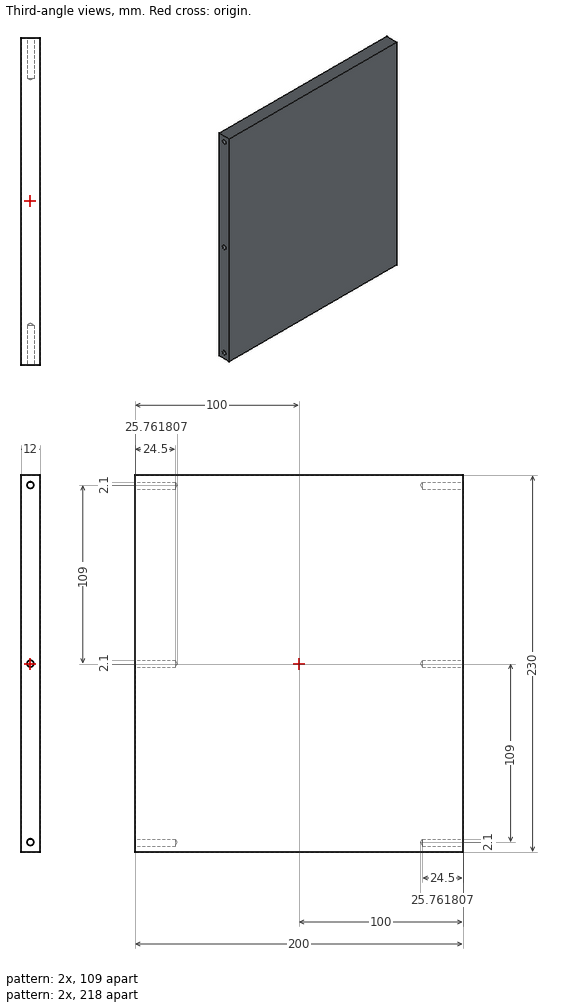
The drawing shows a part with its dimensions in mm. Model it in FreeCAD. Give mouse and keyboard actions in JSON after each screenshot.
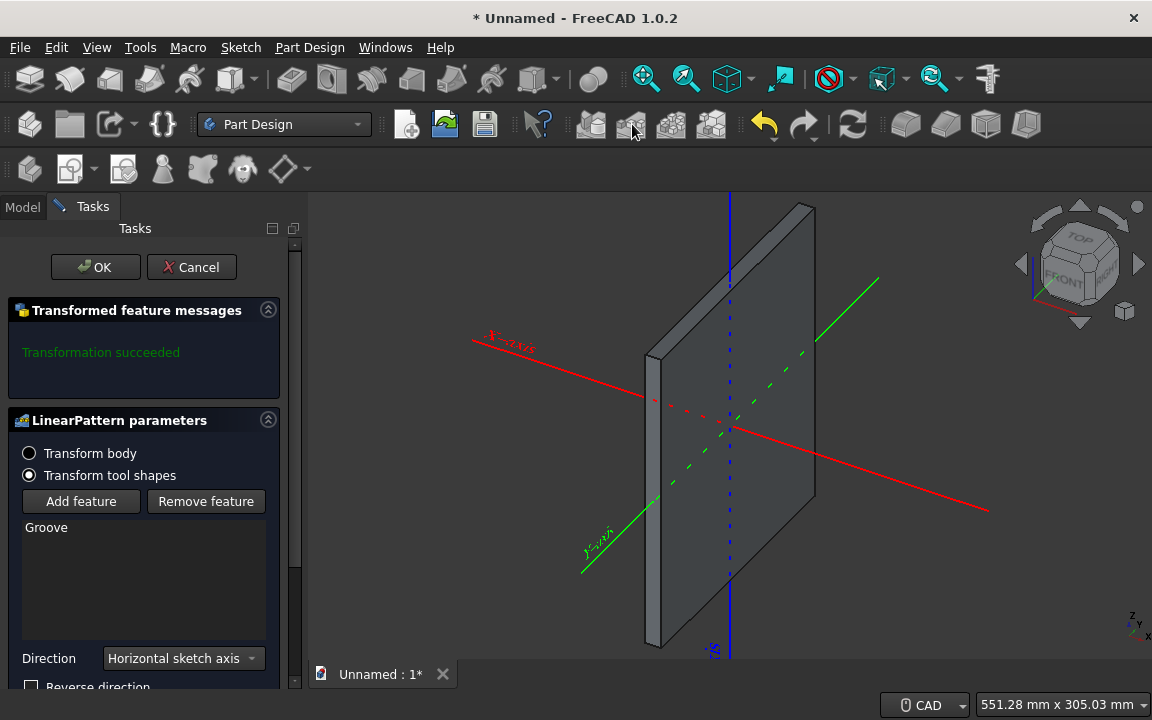
{"action": "left_click", "coordinate": [184, 658]}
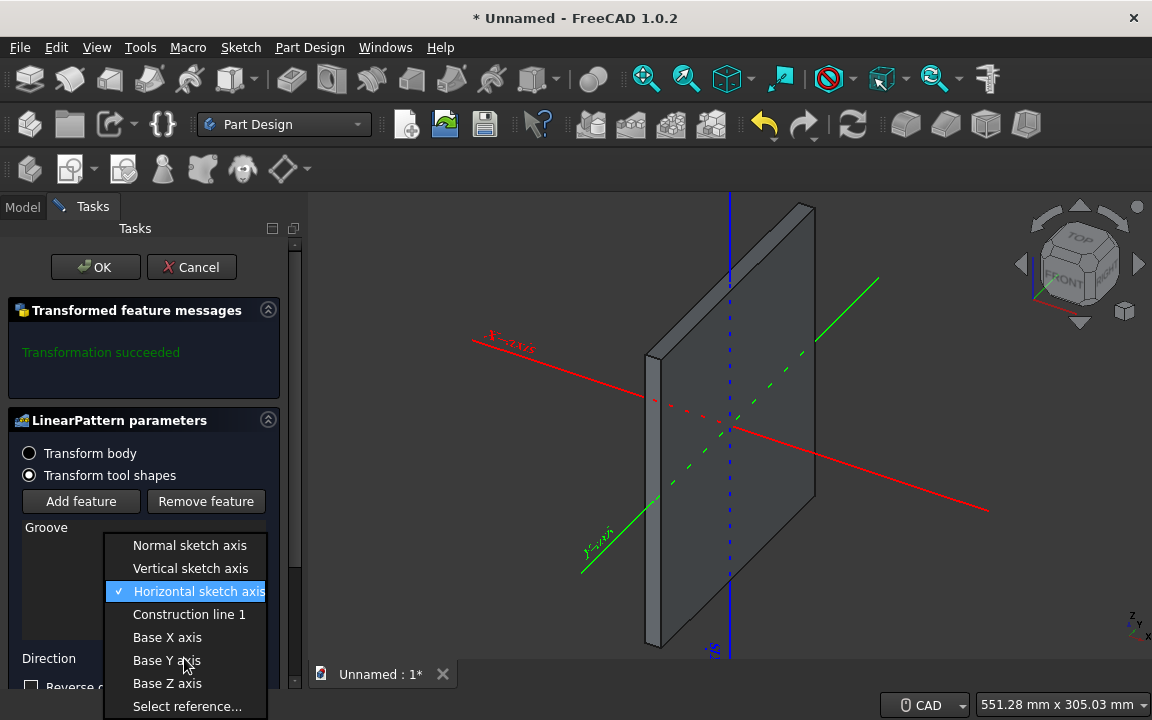
{"action": "left_click", "coordinate": [184, 684]}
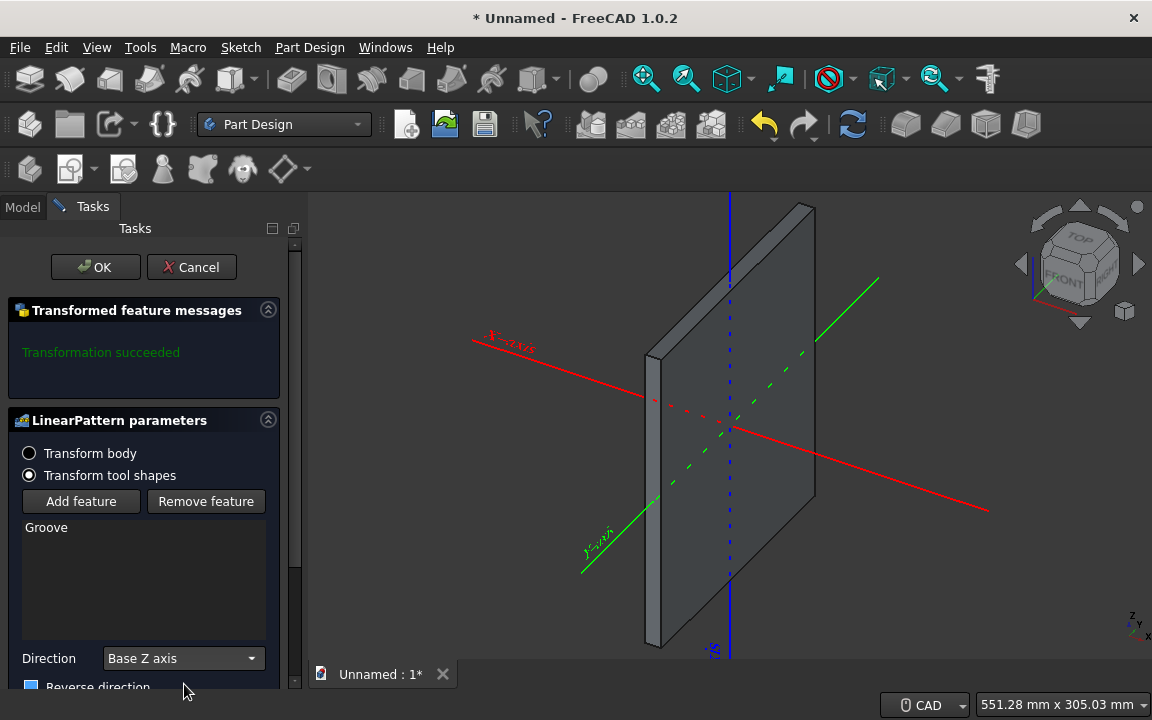
{"action": "scroll", "coordinate": [295, 463], "scroll_direction": "down", "scroll_amount": 2}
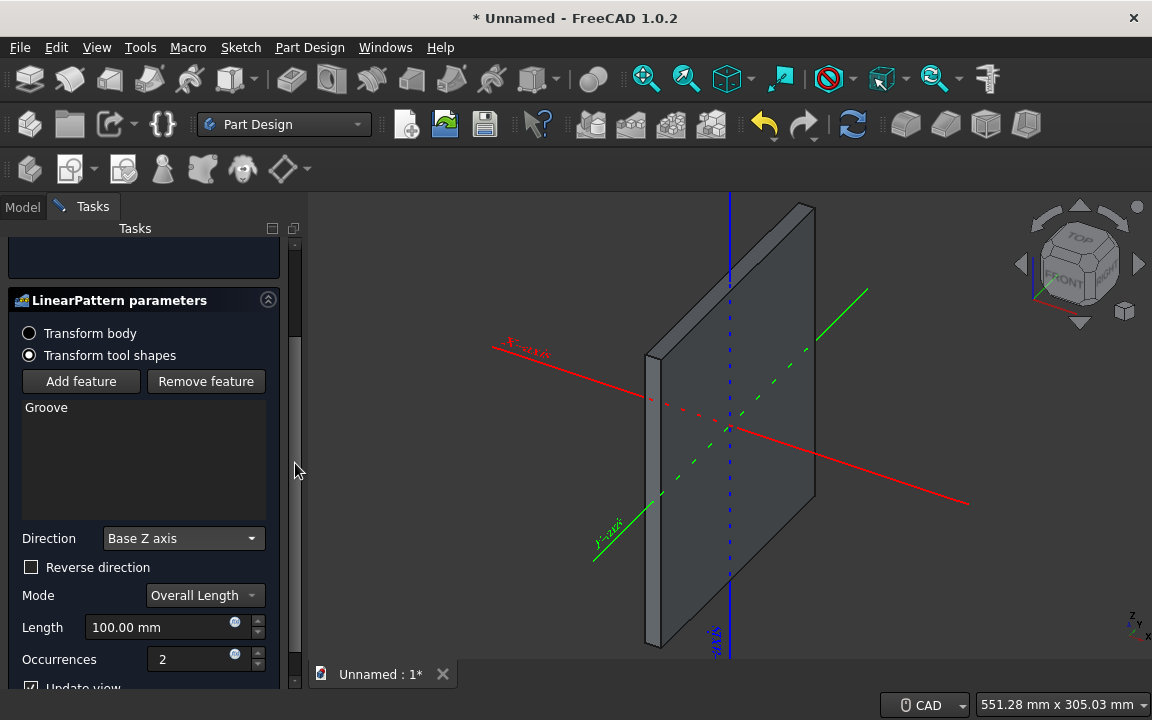
{"action": "left_click", "coordinate": [206, 596]}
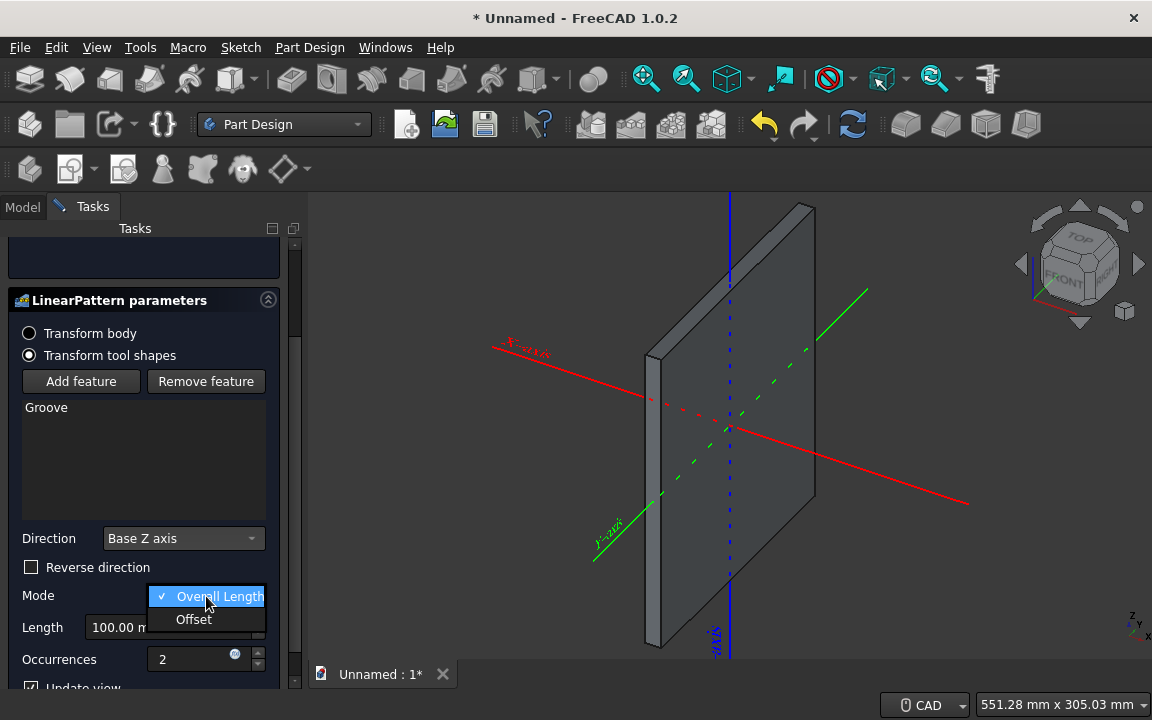
{"action": "left_click", "coordinate": [206, 620]}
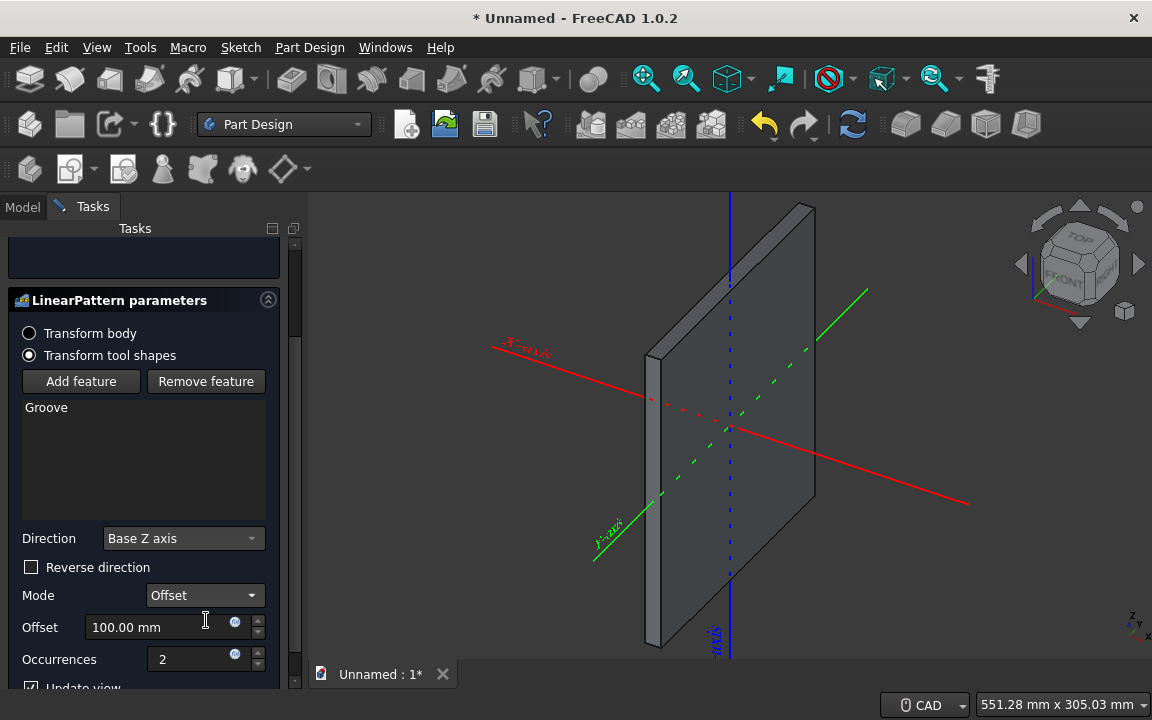
{"action": "triple_click", "coordinate": [168, 627]}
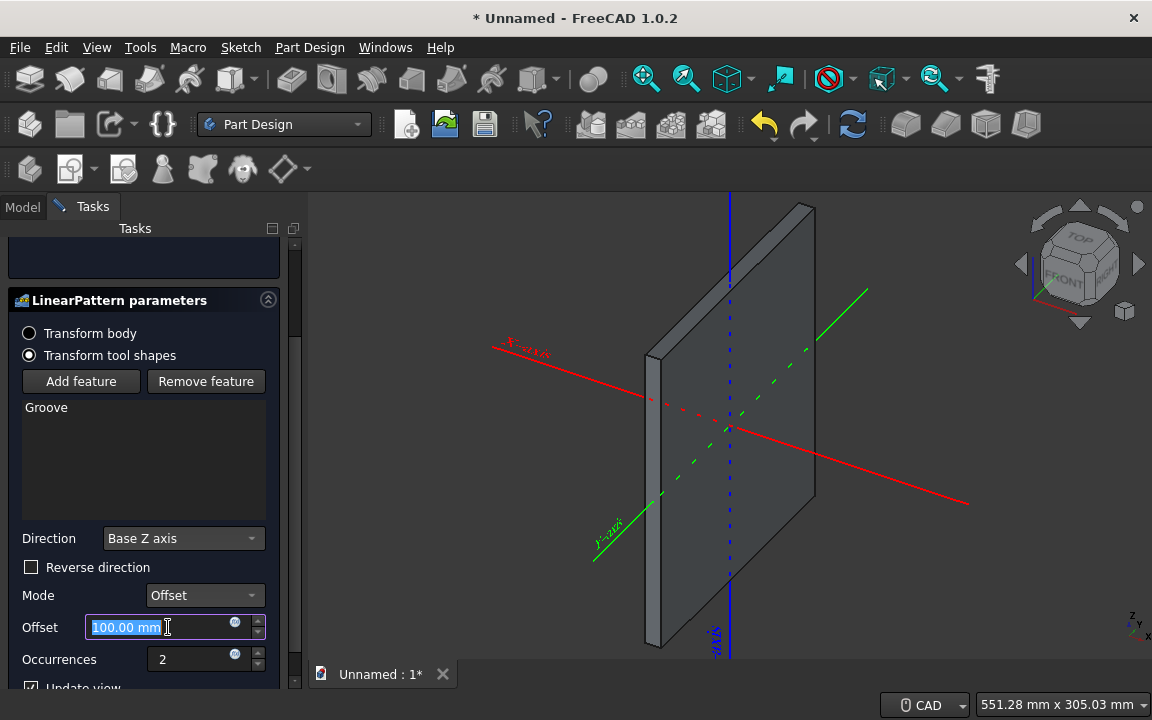
{"action": "type", "text": "109"}
{"action": "key", "text": "Tab"}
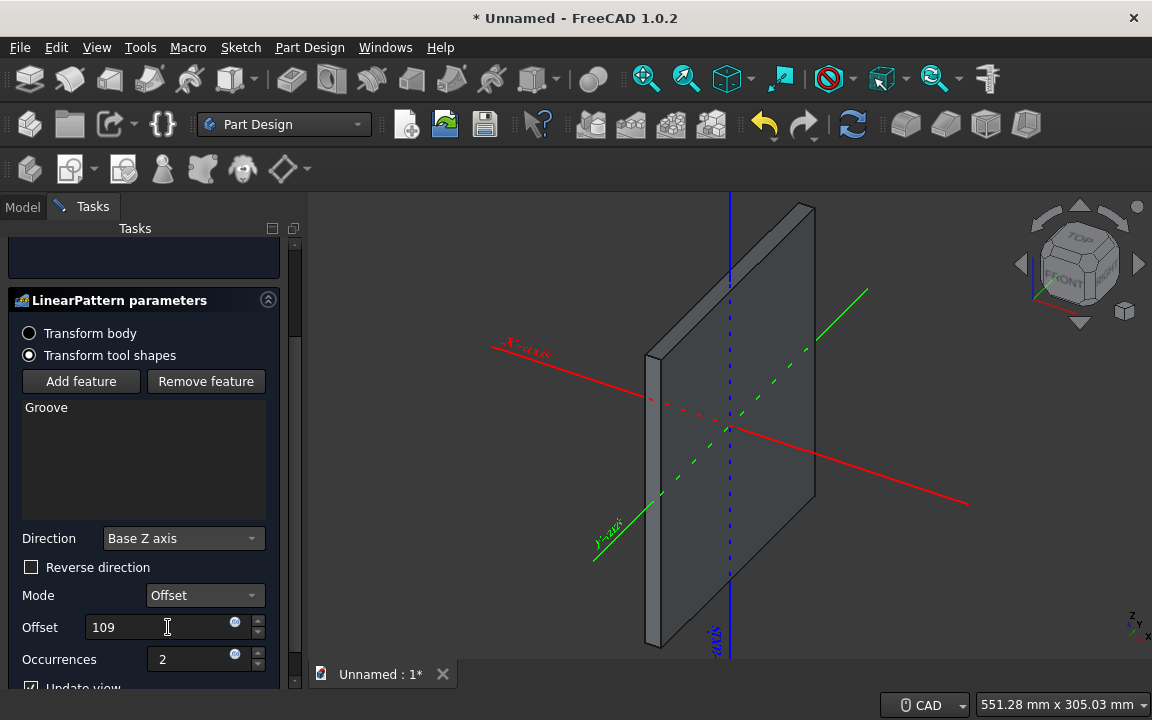
{"action": "triple_click", "coordinate": [198, 659]}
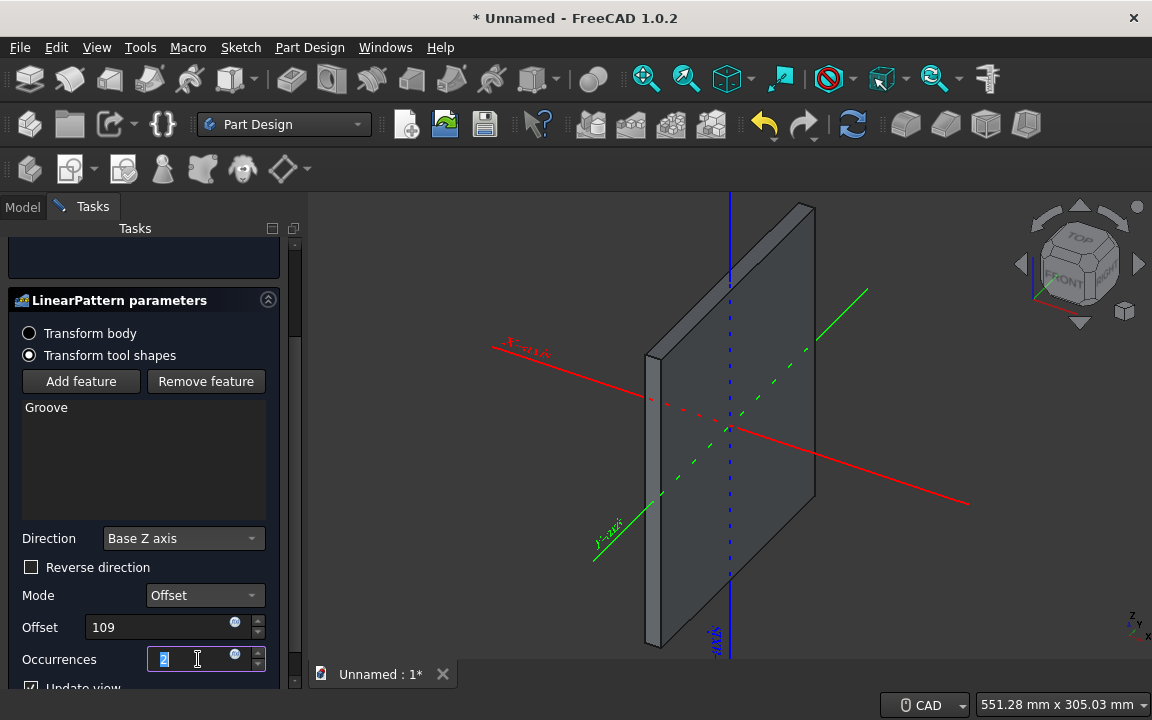
{"action": "type", "text": "2"}
{"action": "key", "text": "Tab"}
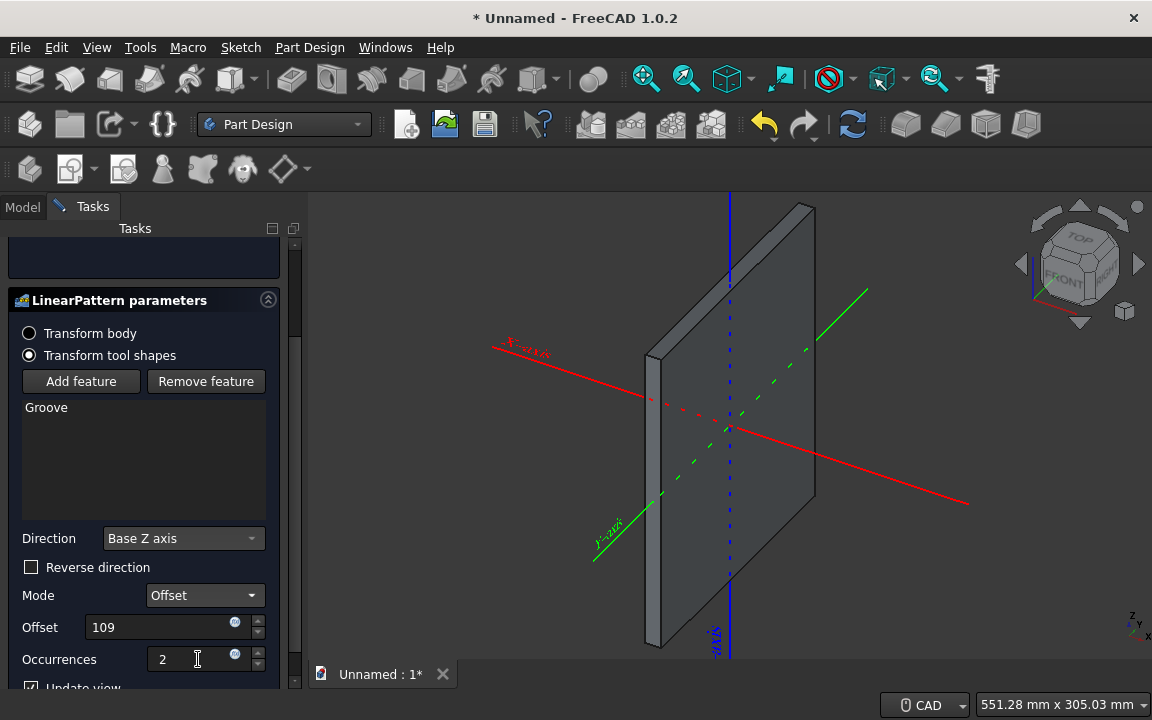
{"action": "scroll", "coordinate": [295, 463], "scroll_direction": "up", "scroll_amount": 3}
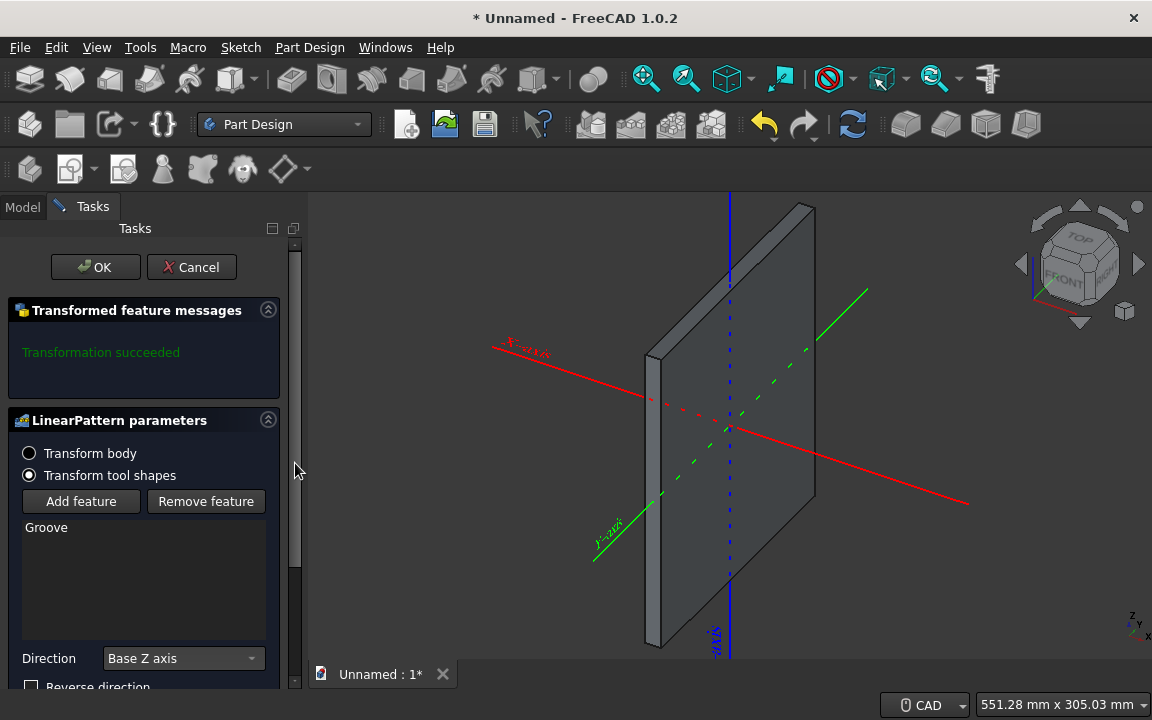
{"action": "left_click", "coordinate": [96, 267]}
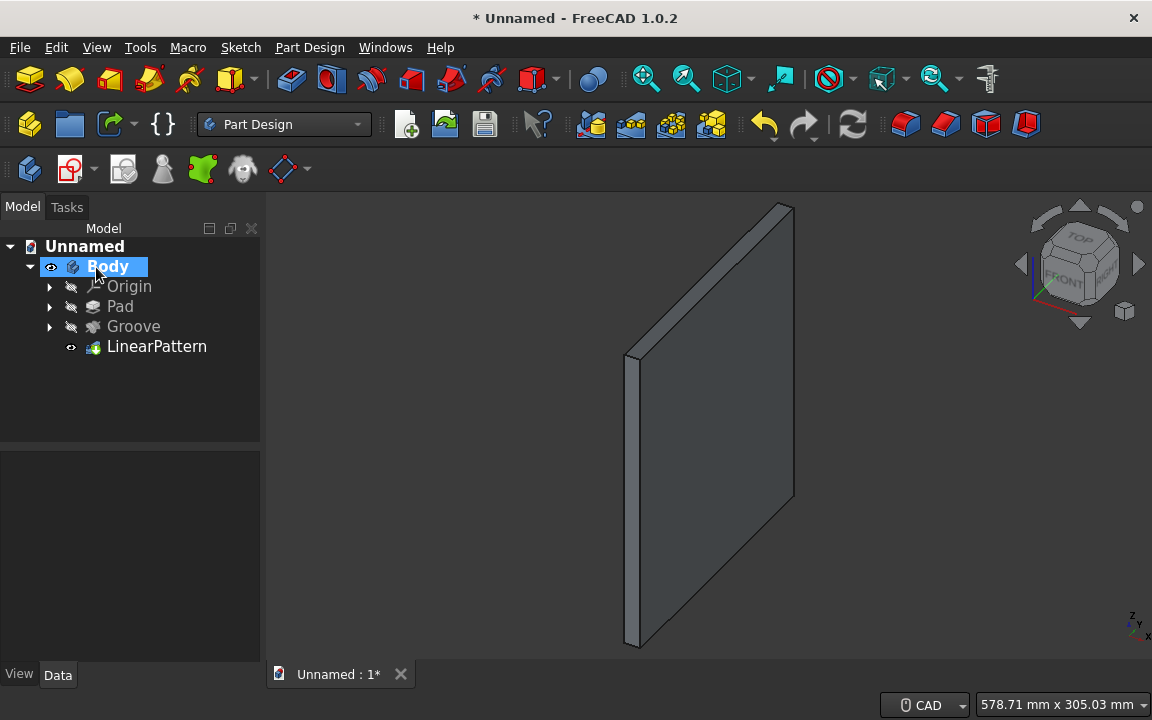
{"action": "left_click", "coordinate": [116, 327]}